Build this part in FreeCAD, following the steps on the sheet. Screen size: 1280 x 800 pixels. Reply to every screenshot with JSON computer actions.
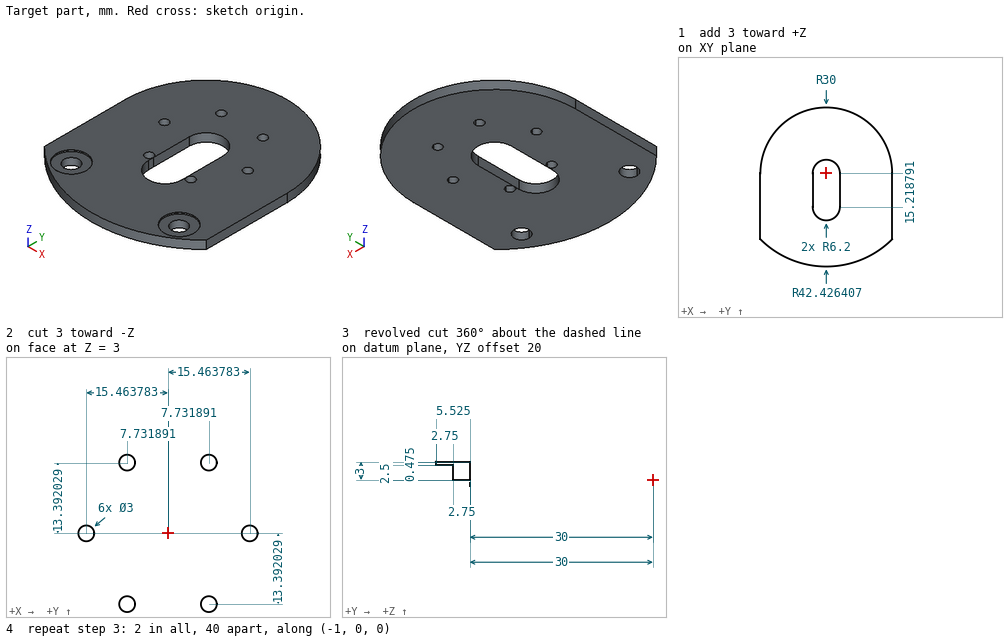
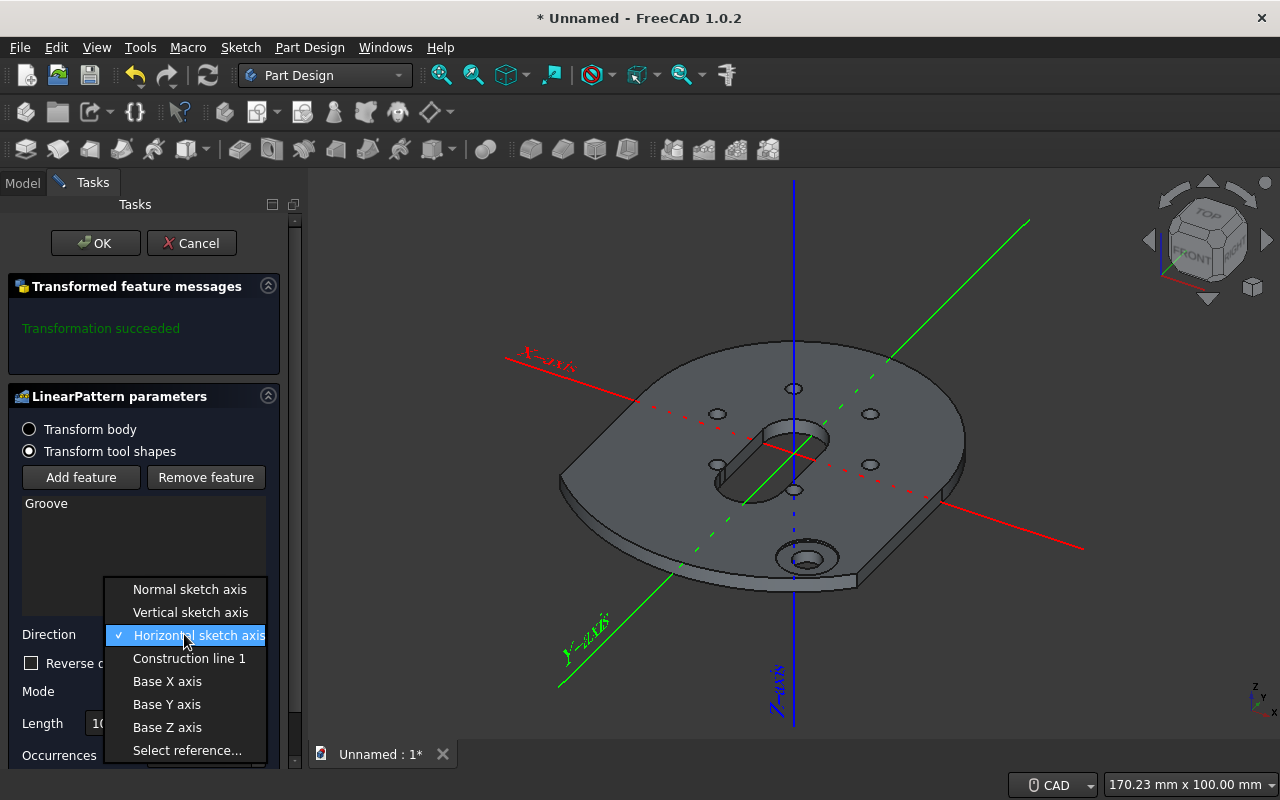
{"action": "left_click", "coordinate": [184, 682]}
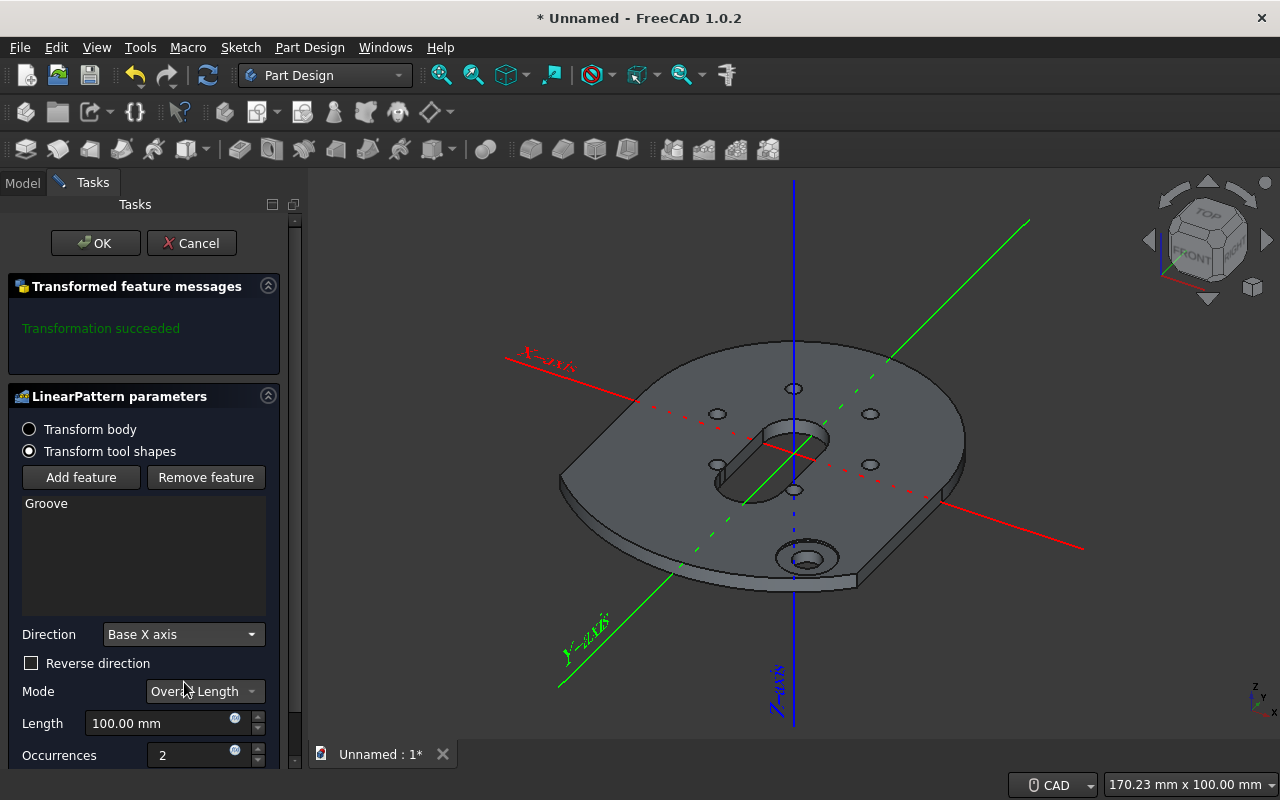
{"action": "left_click", "coordinate": [206, 692]}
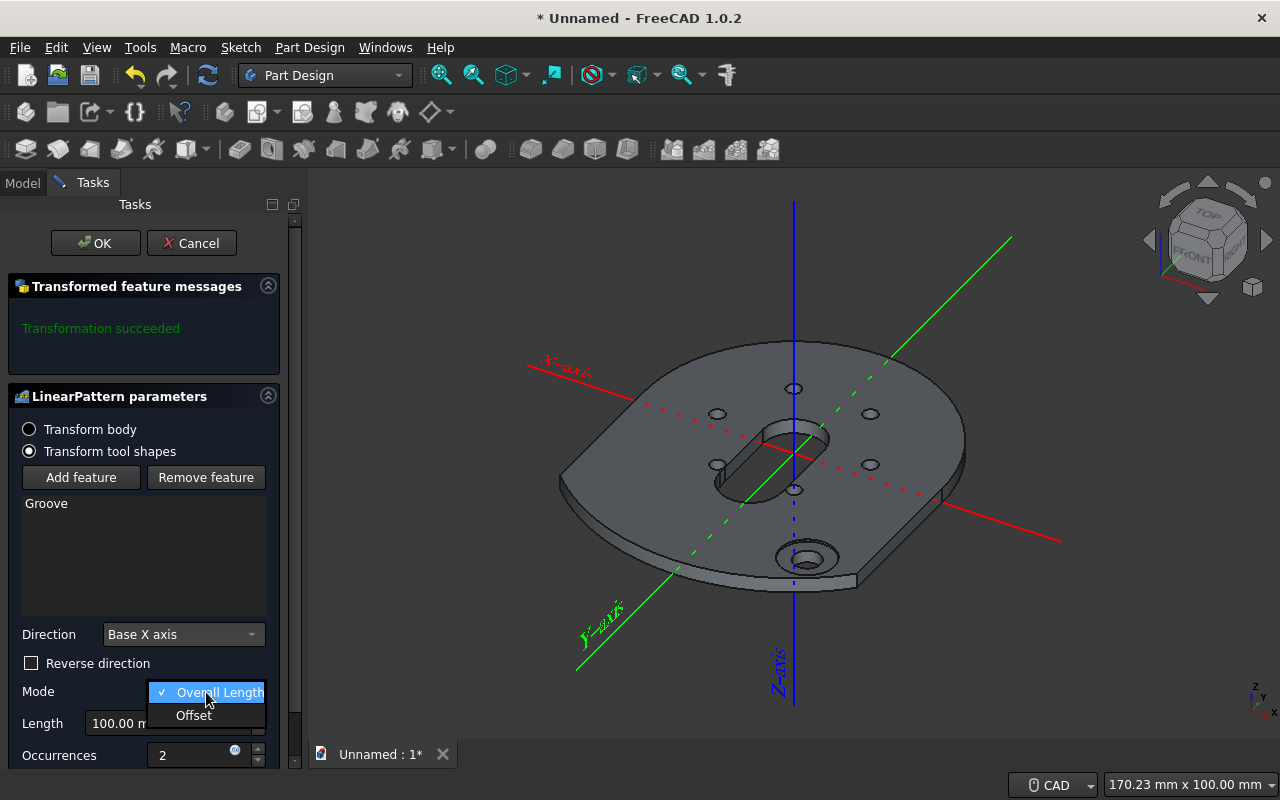
{"action": "left_click", "coordinate": [206, 716]}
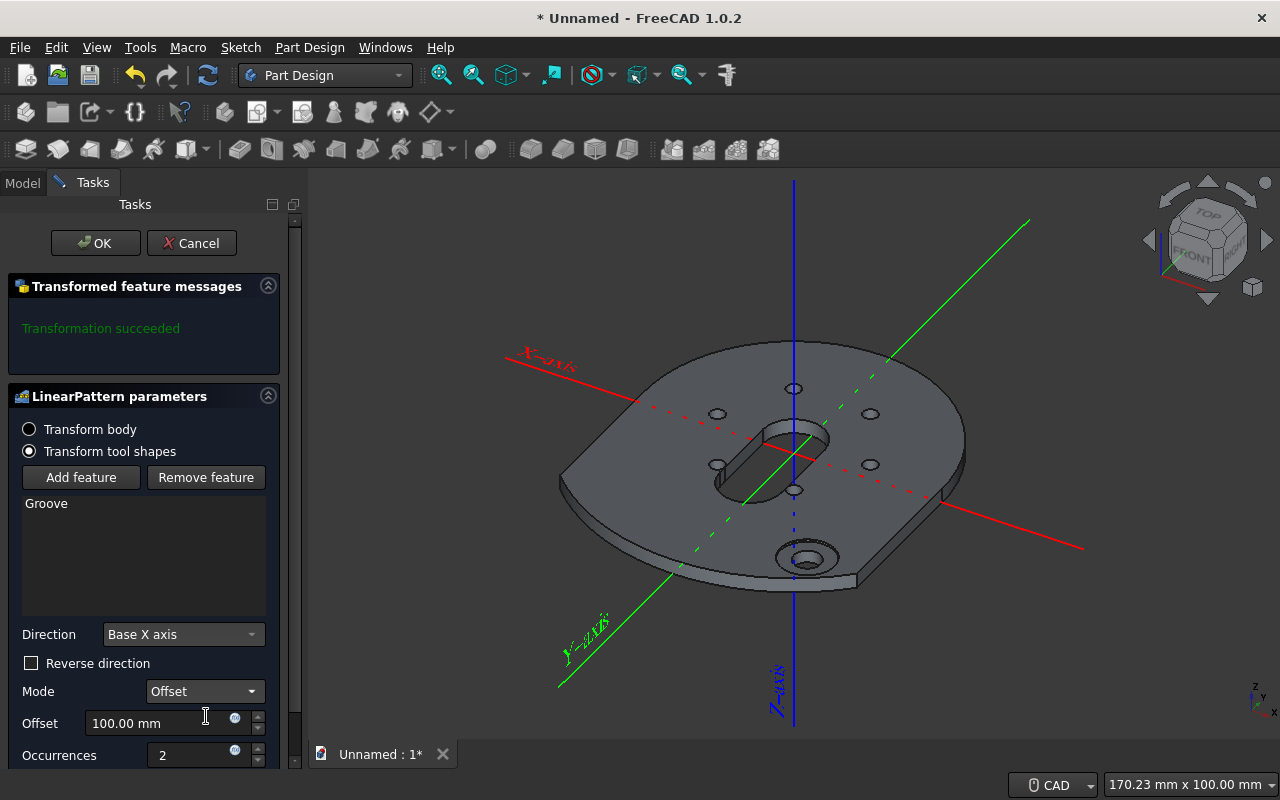
{"action": "triple_click", "coordinate": [168, 723]}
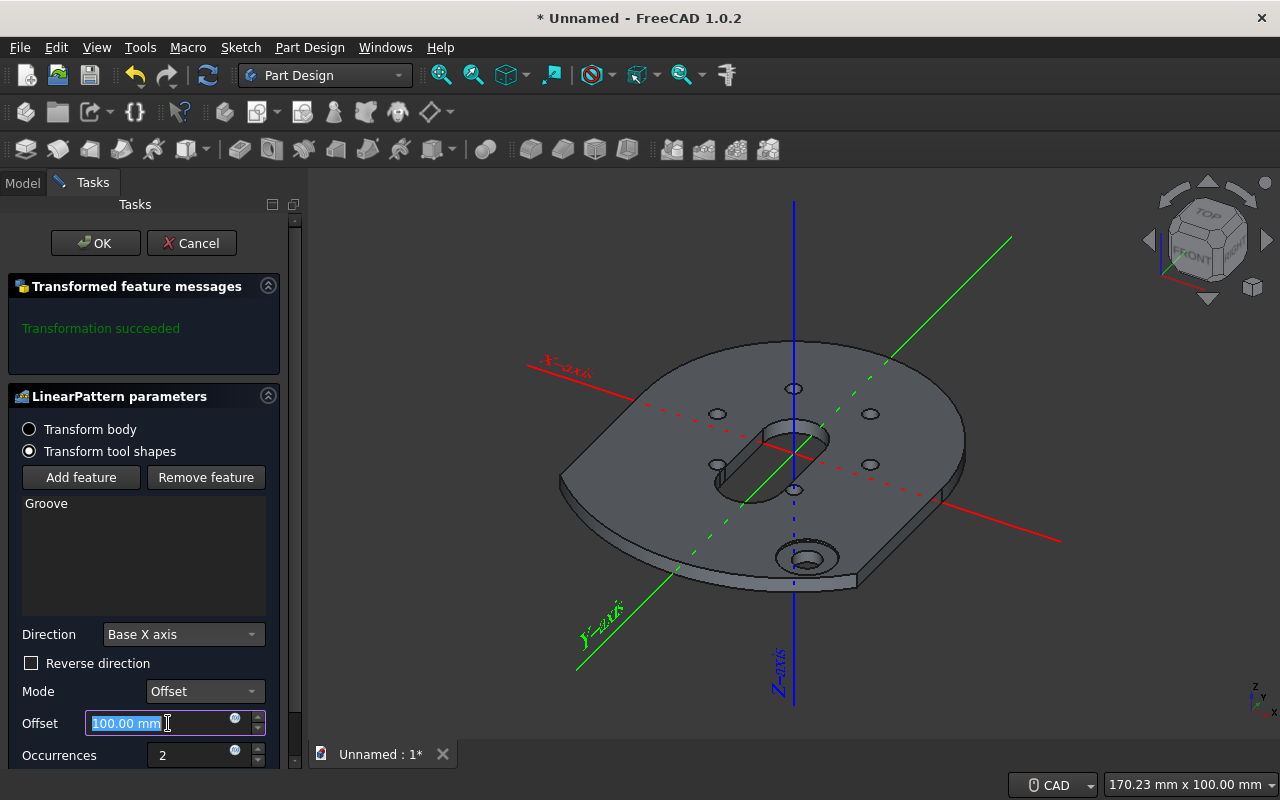
{"action": "type", "text": "40"}
{"action": "key", "text": "Tab"}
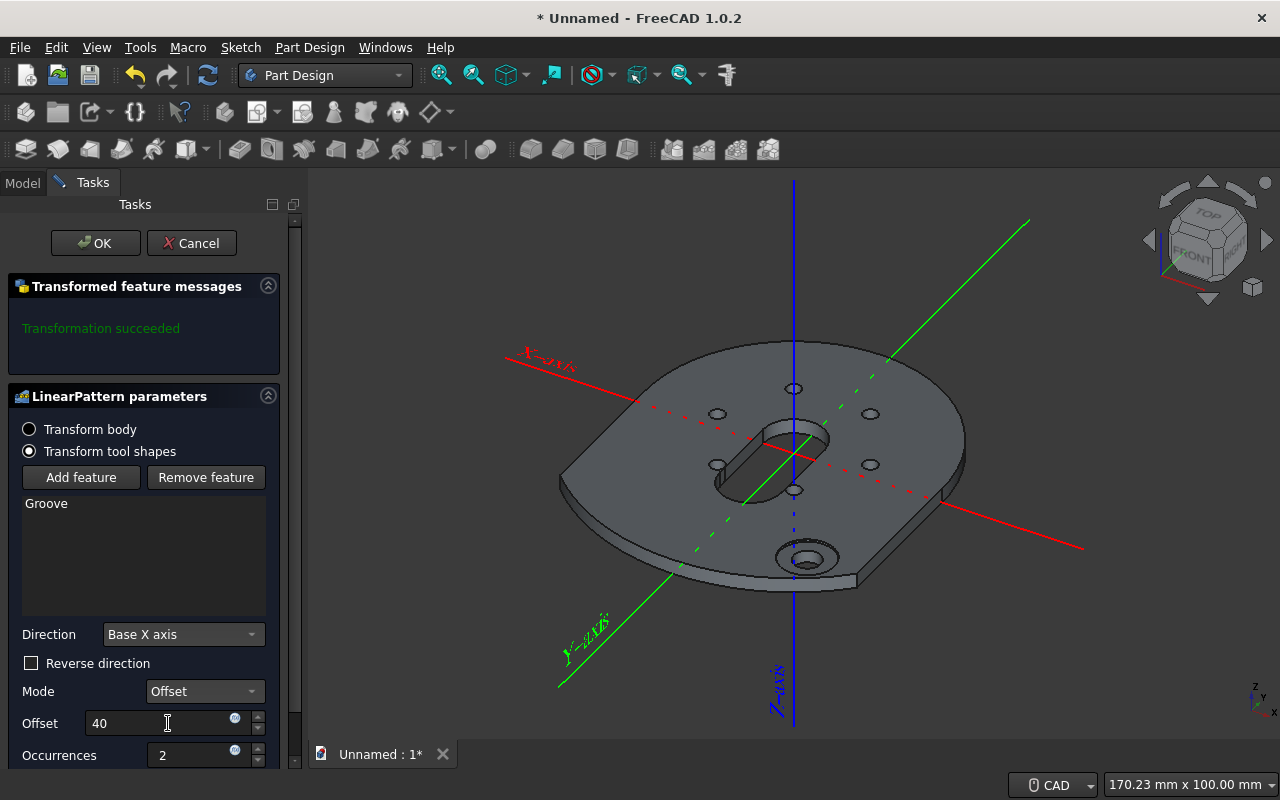
{"action": "triple_click", "coordinate": [198, 755]}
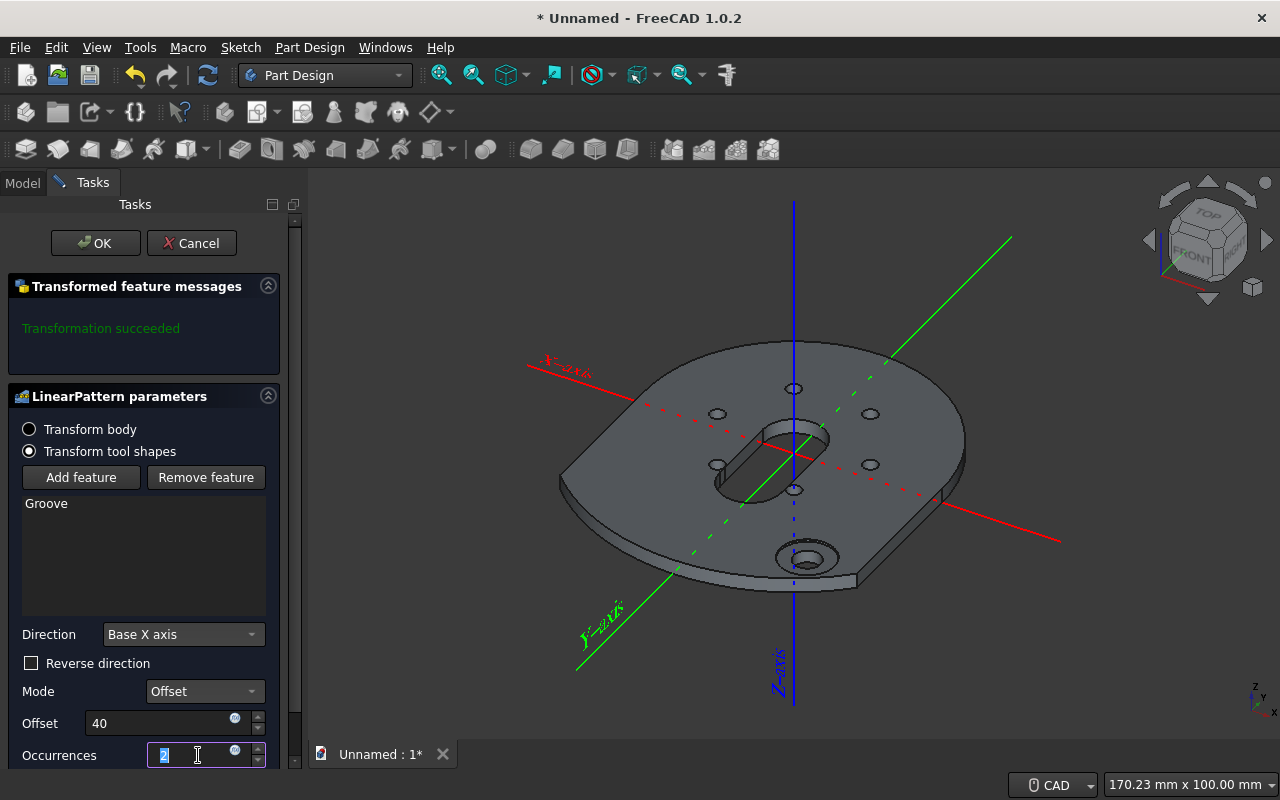
{"action": "type", "text": "2"}
{"action": "key", "text": "Tab"}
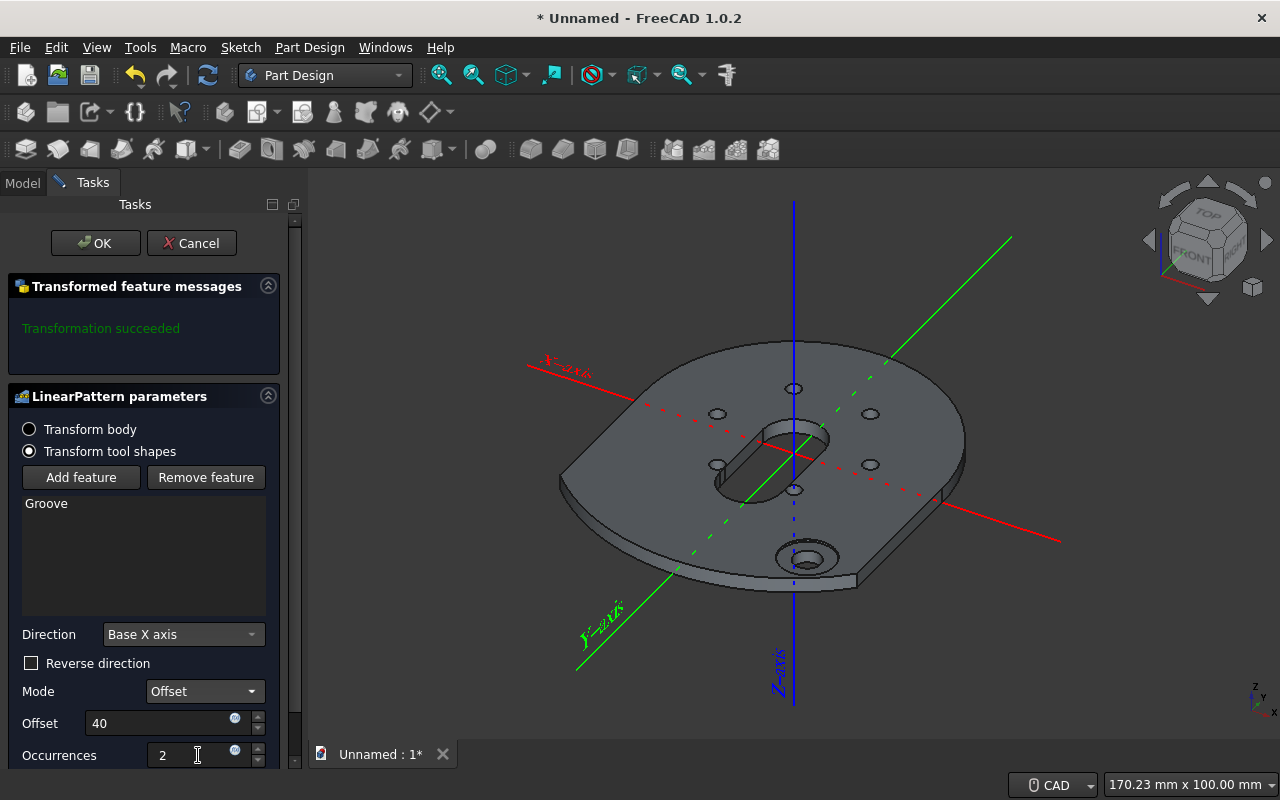
{"action": "left_click", "coordinate": [30, 663]}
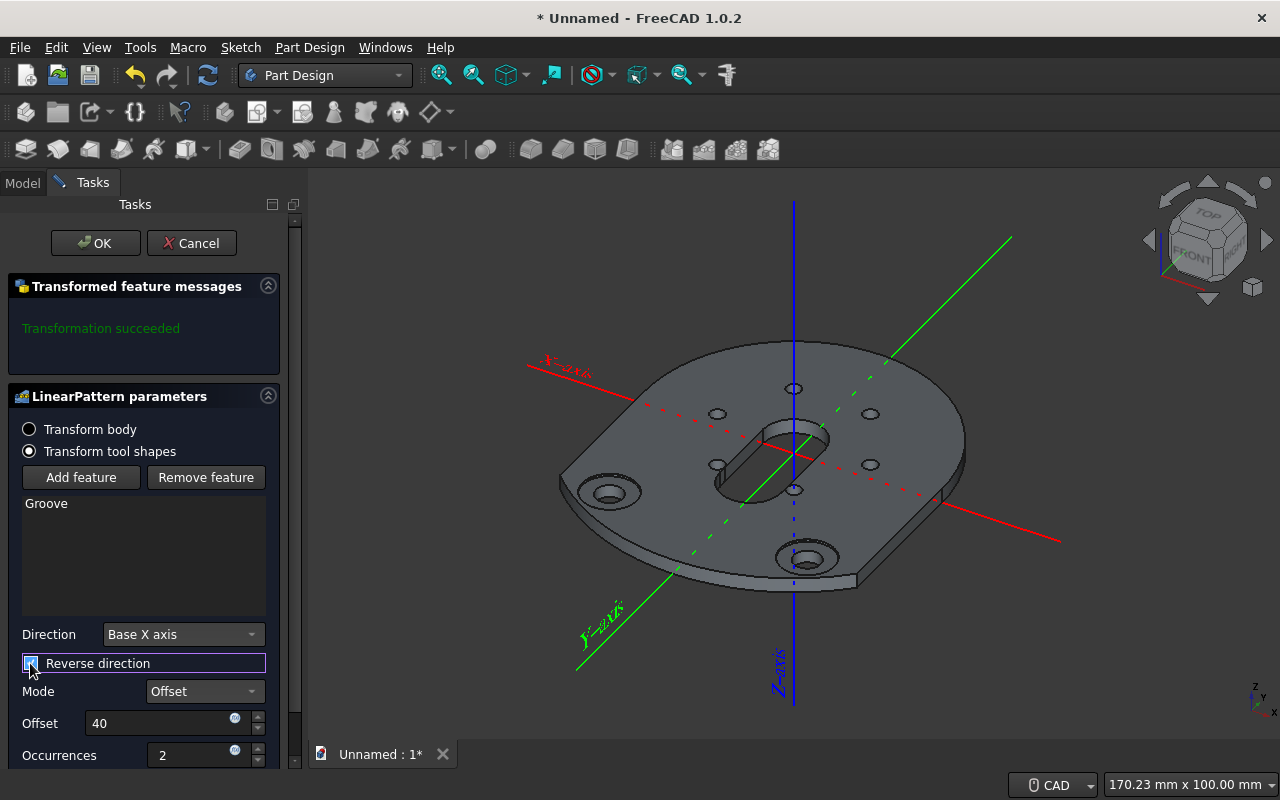
{"action": "left_click", "coordinate": [96, 243]}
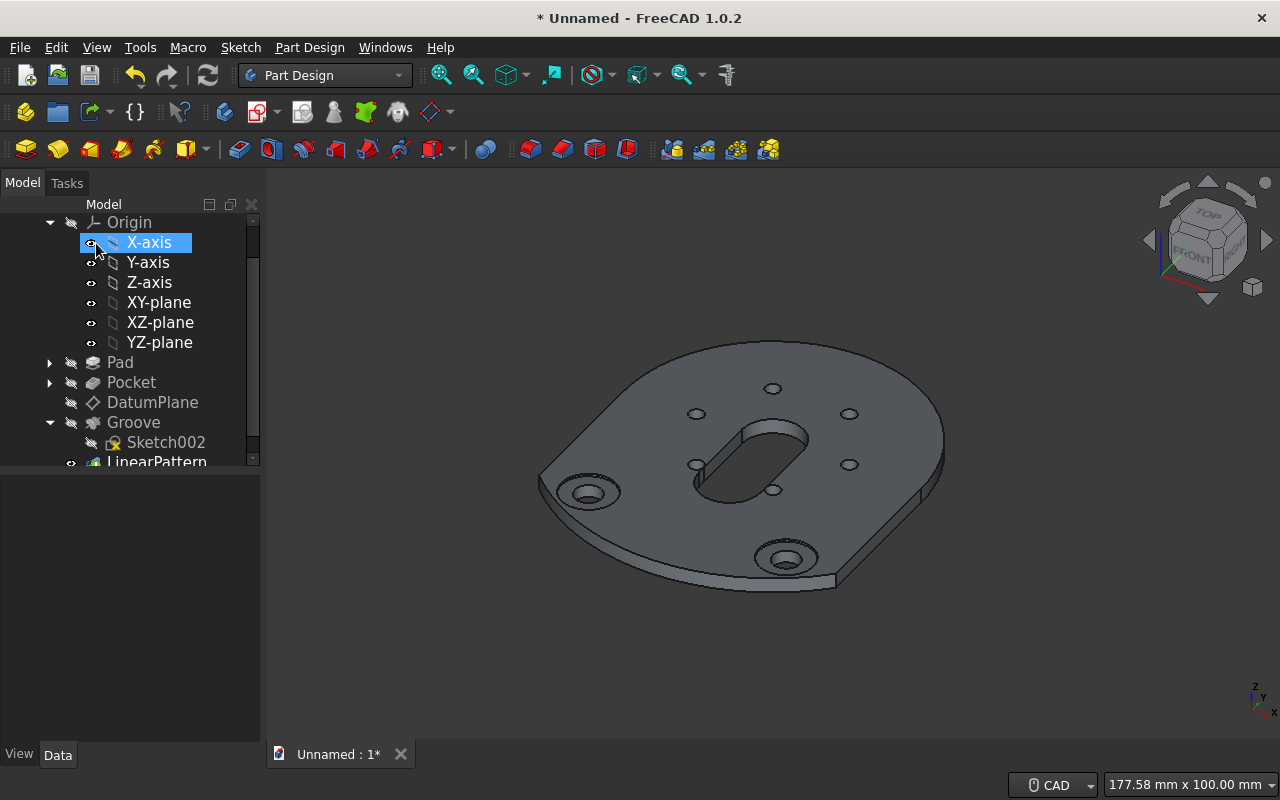
{"action": "key", "text": "0"}